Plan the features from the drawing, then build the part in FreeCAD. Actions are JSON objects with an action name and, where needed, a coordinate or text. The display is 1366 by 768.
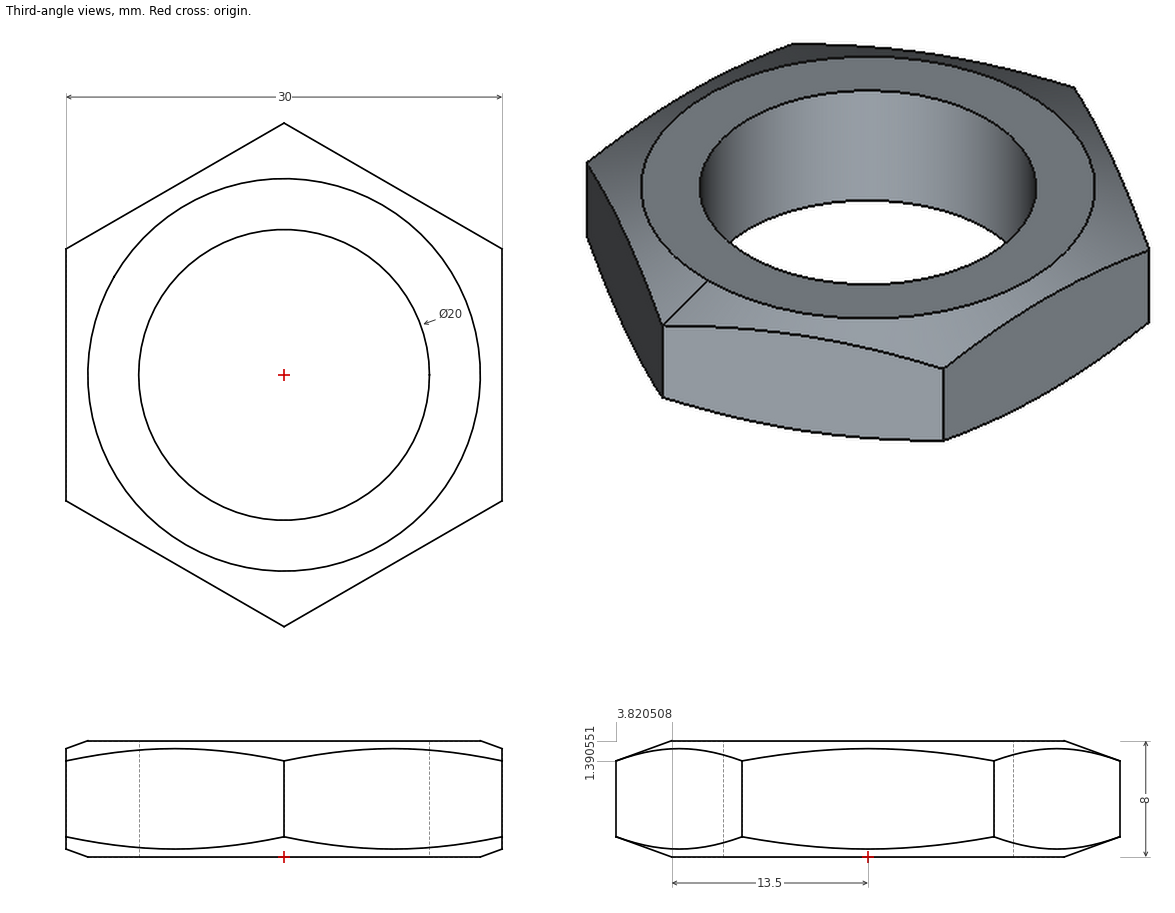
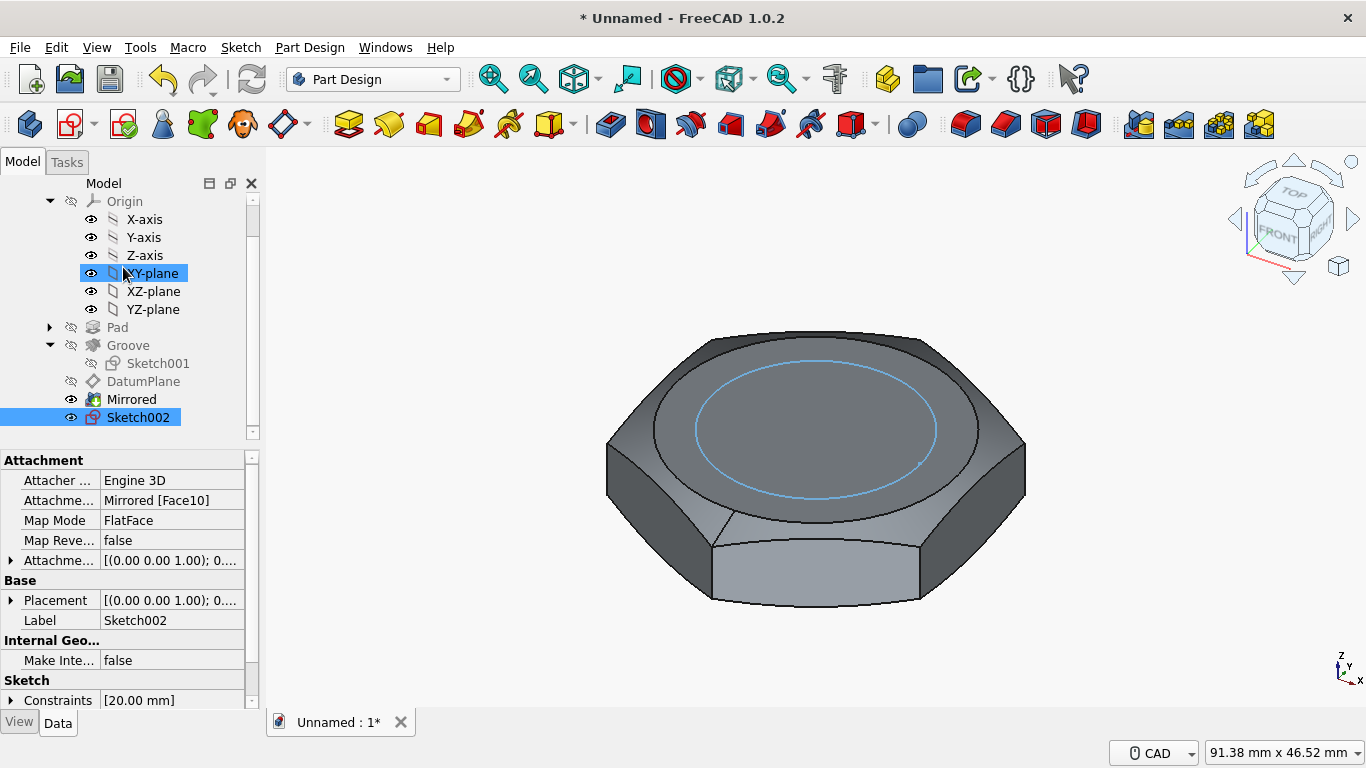
{"action": "left_click", "coordinate": [612, 124]}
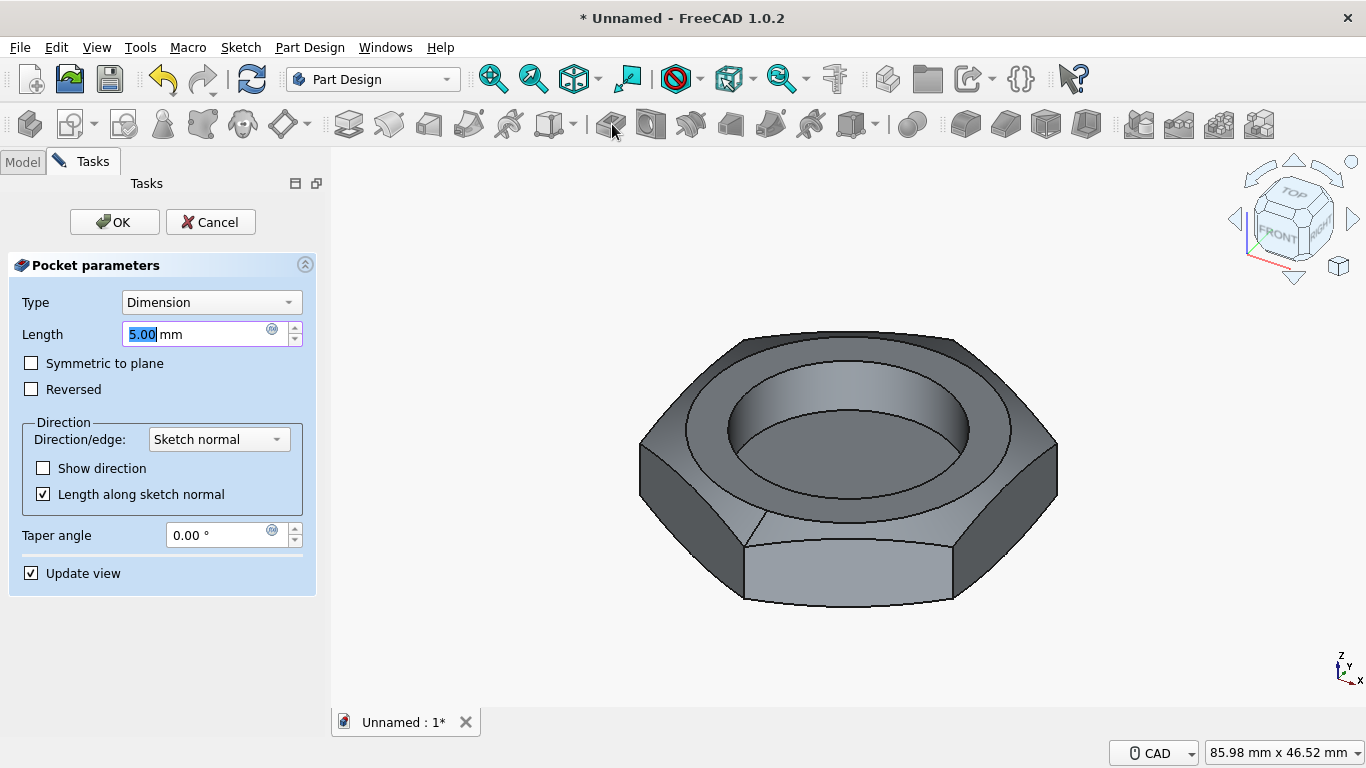
{"action": "left_click", "coordinate": [212, 302]}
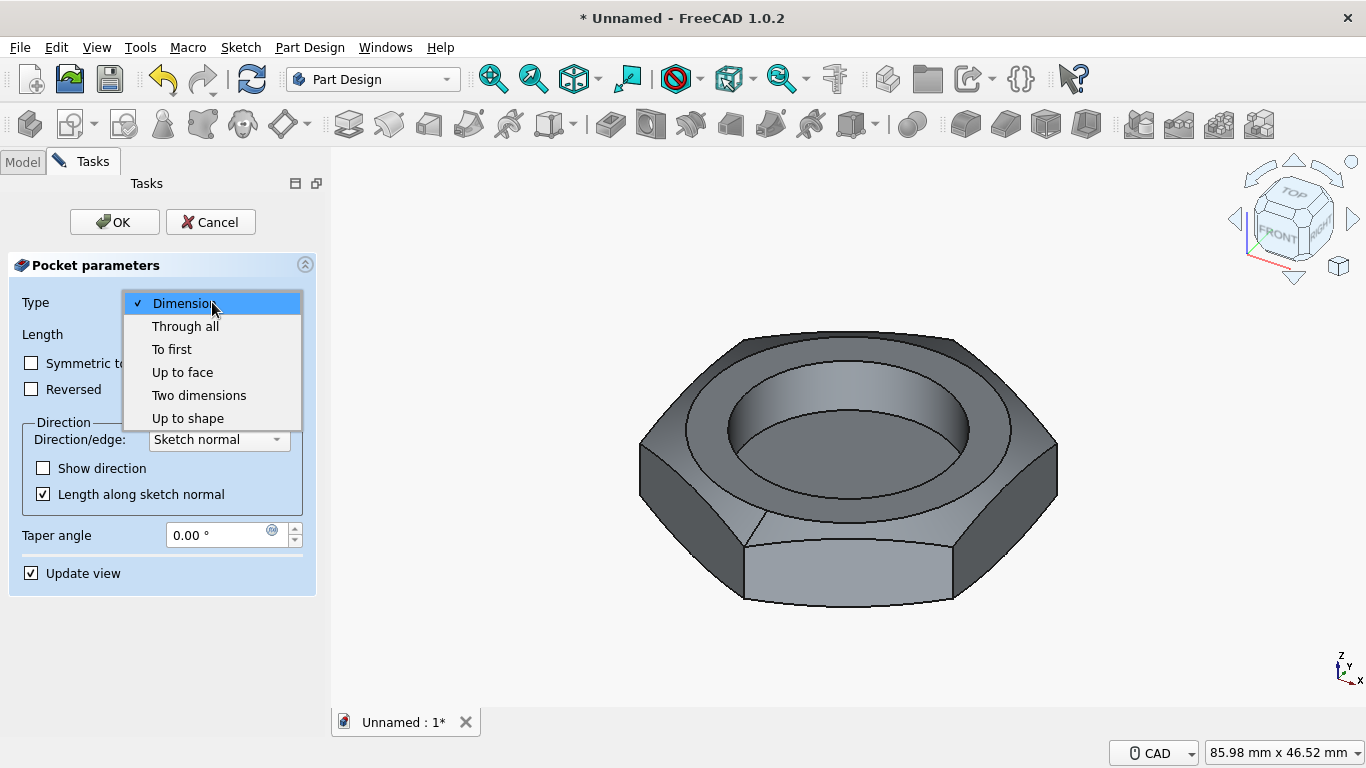
{"action": "left_click", "coordinate": [212, 326]}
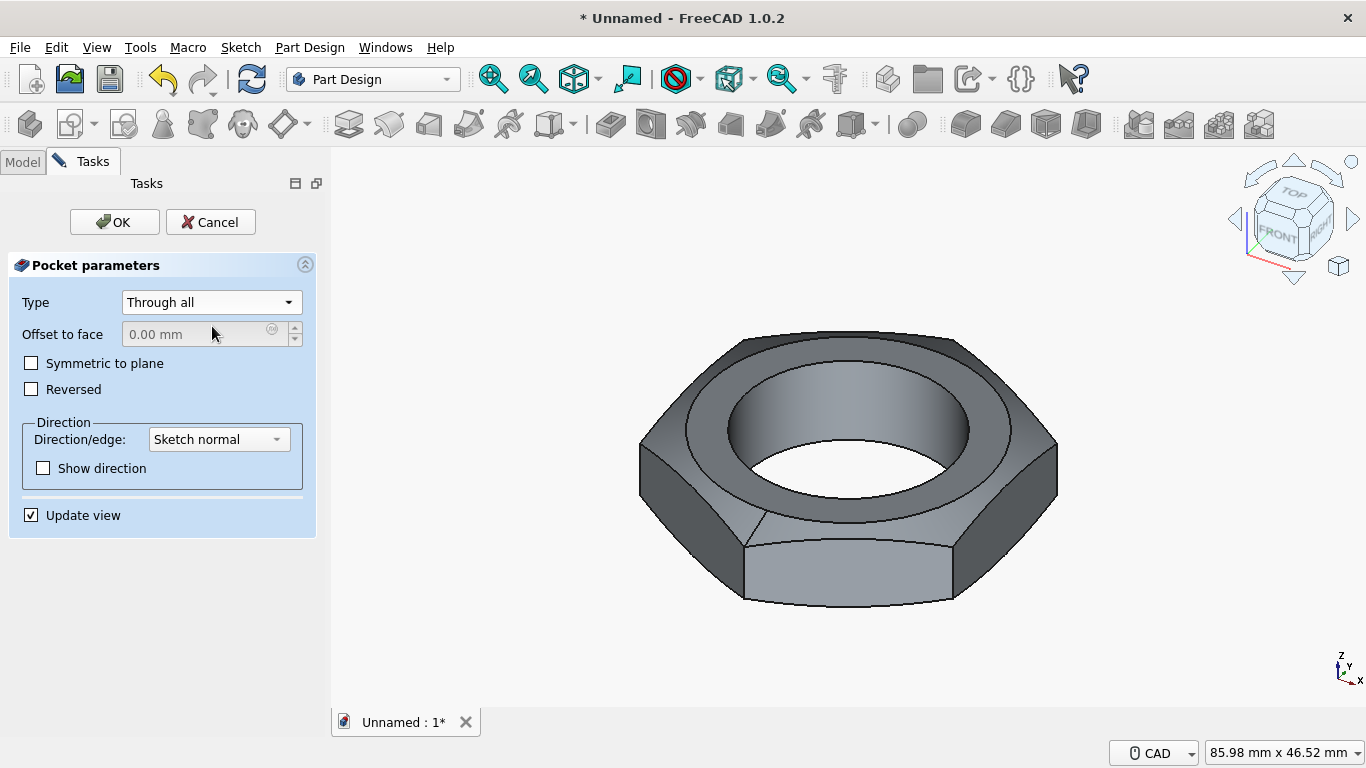
{"action": "left_click", "coordinate": [115, 222]}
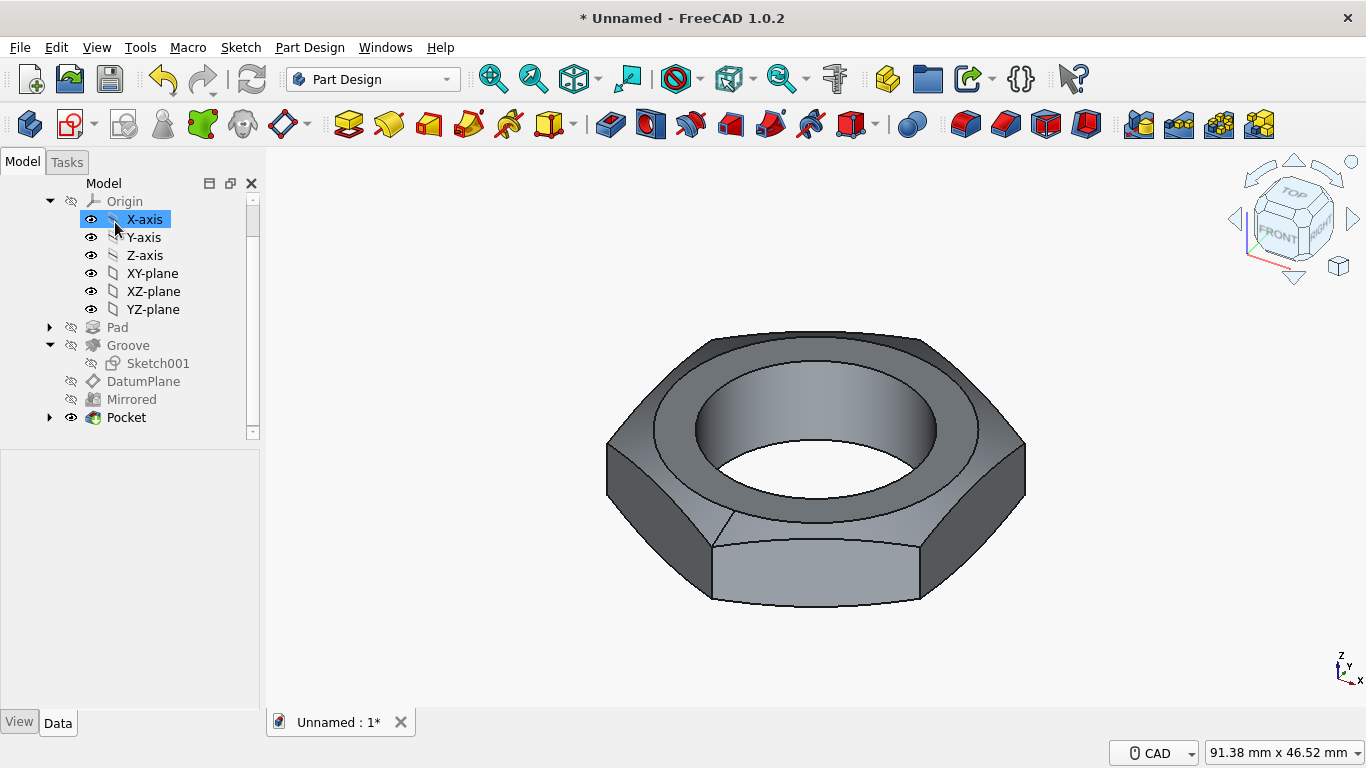
{"action": "key", "text": "0"}